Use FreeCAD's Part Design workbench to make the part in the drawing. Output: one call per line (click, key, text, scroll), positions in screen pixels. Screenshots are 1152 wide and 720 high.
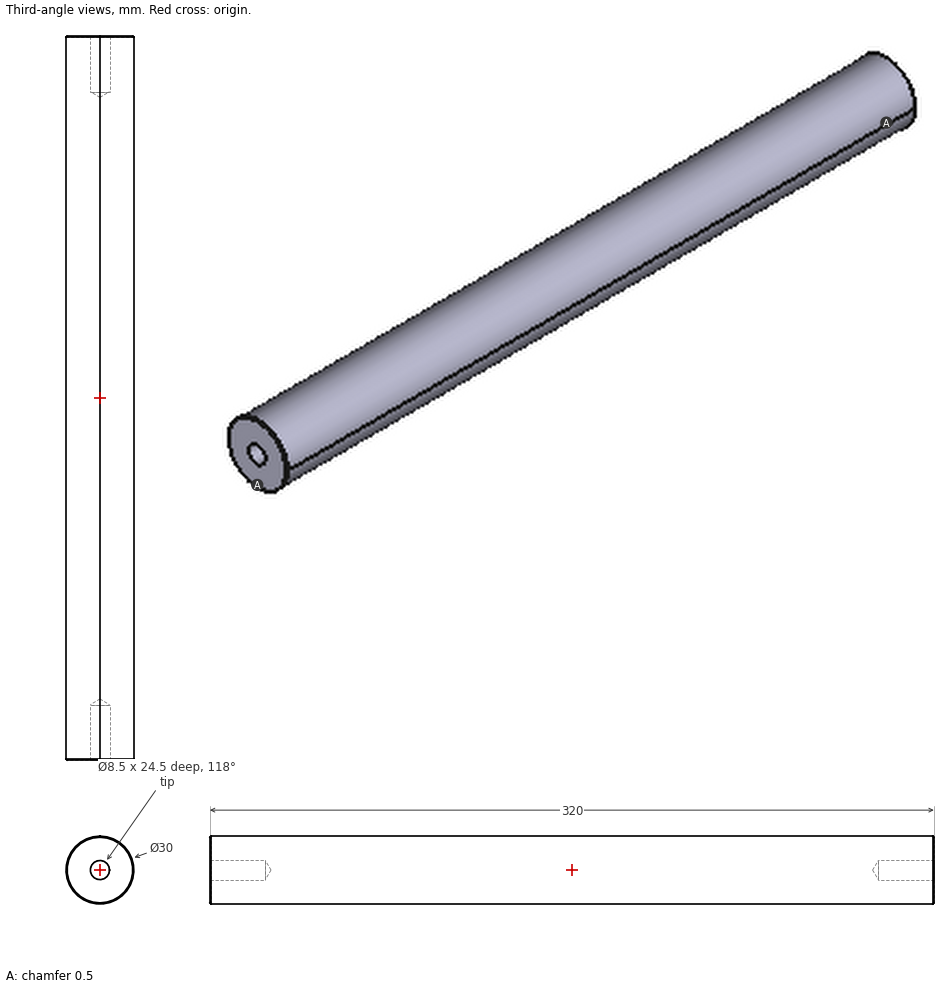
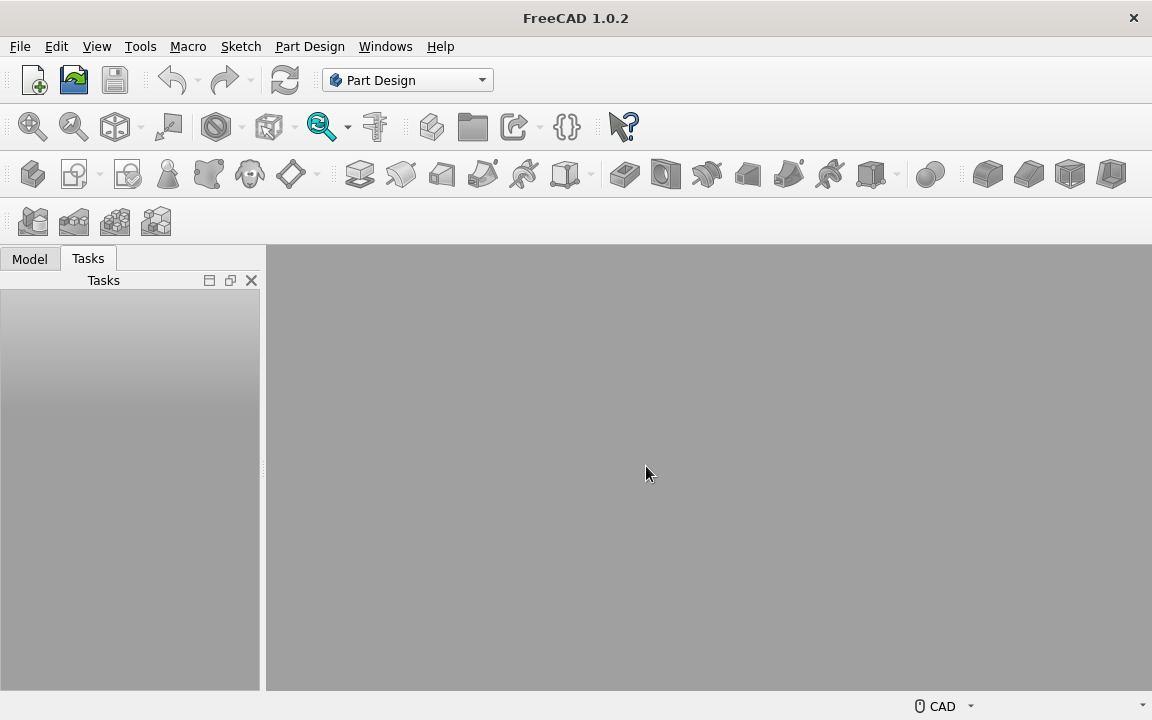
key(ctrl+n)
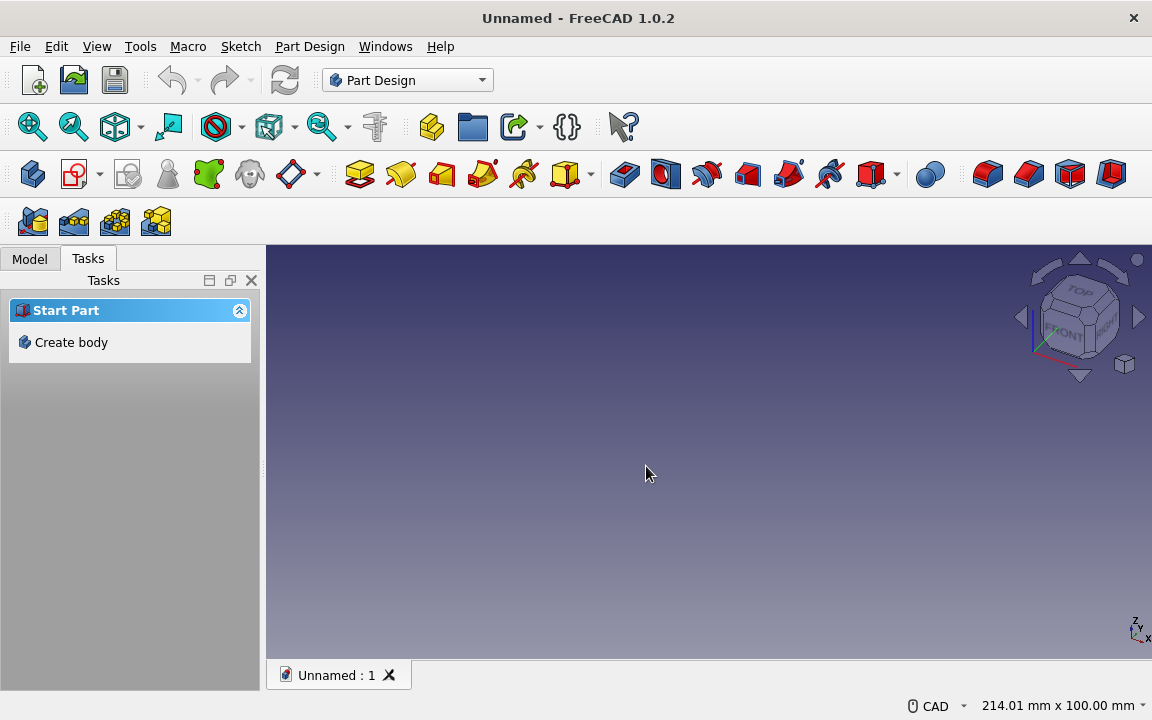
click(74, 174)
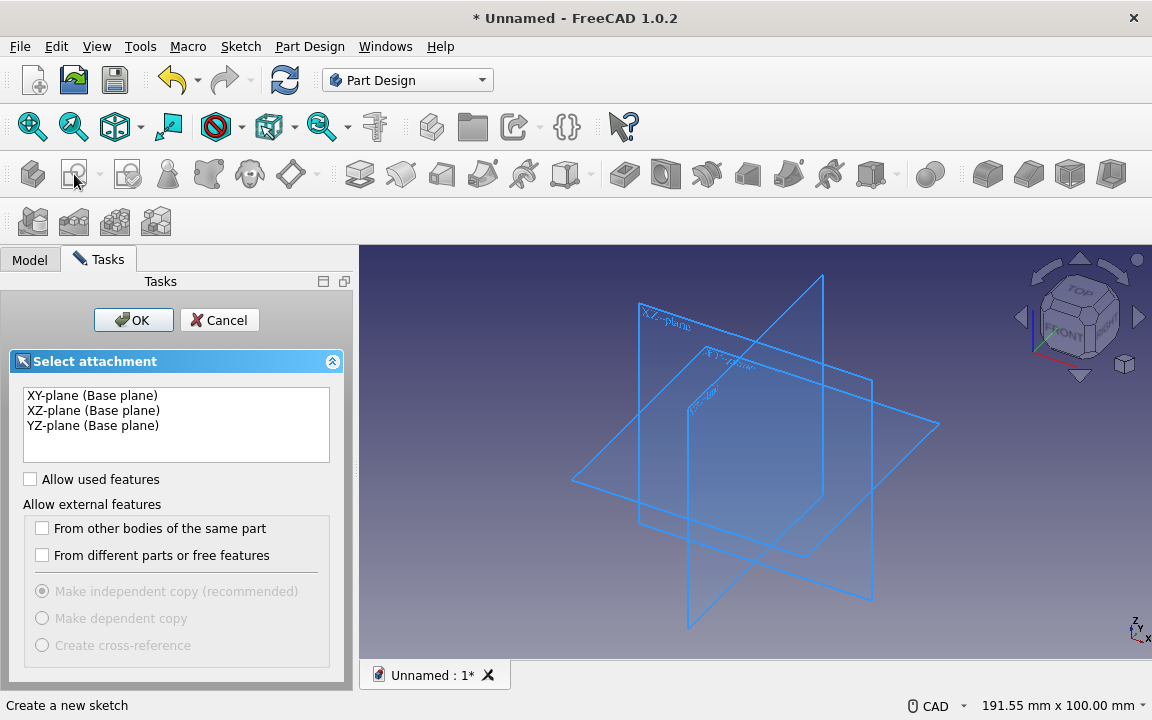
click(84, 410)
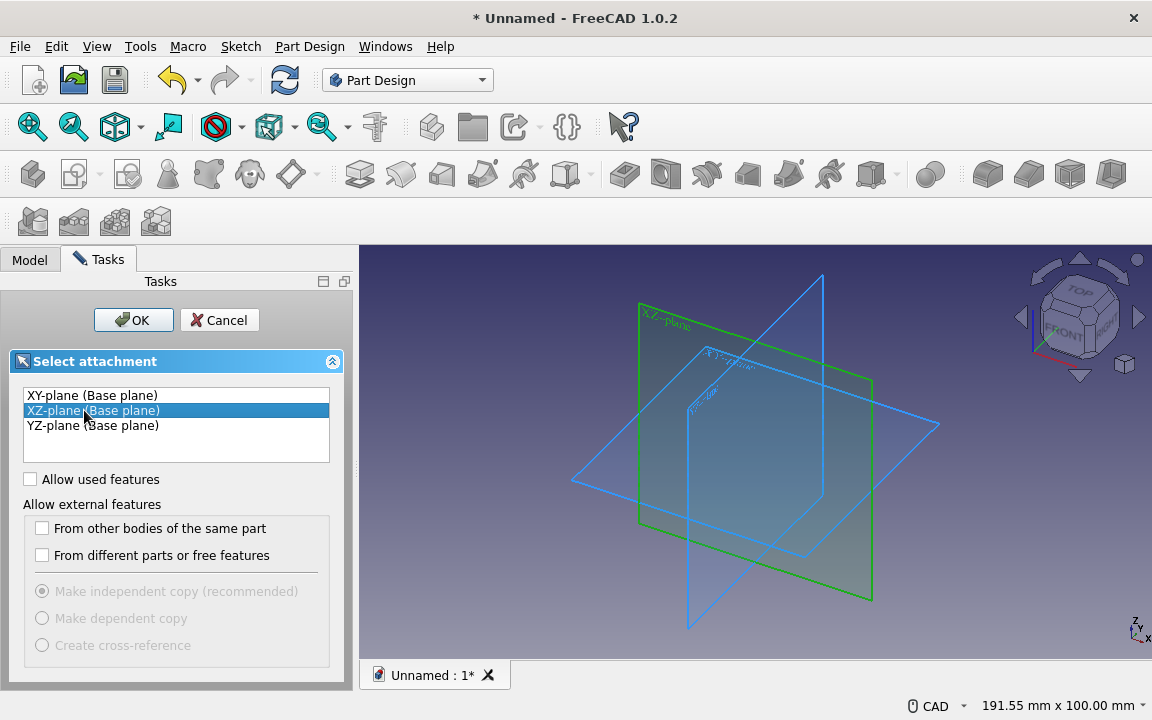
click(134, 320)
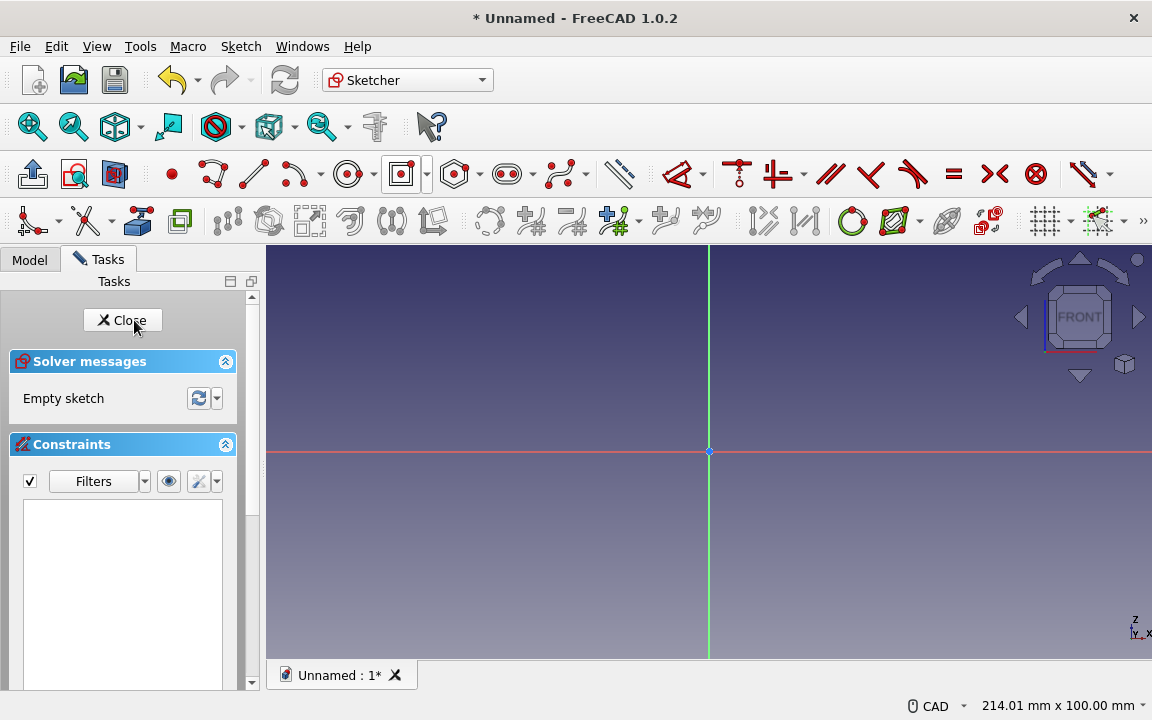
scroll(765, 452, up, 4)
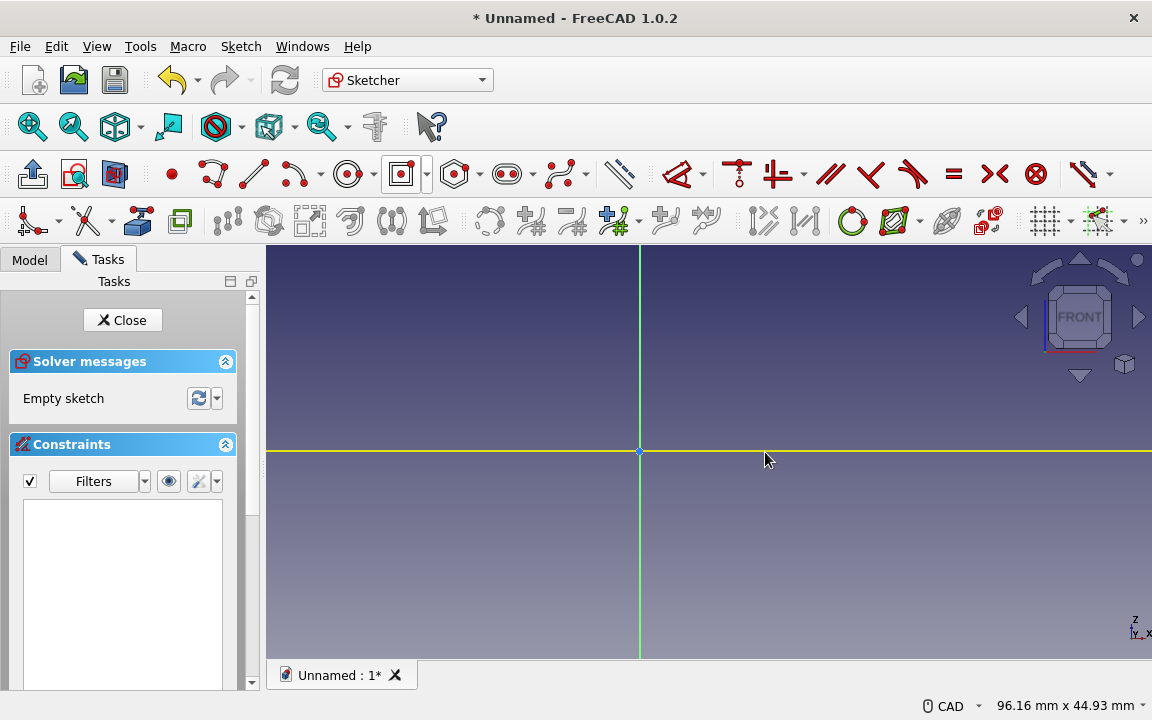
key(g)
key(c)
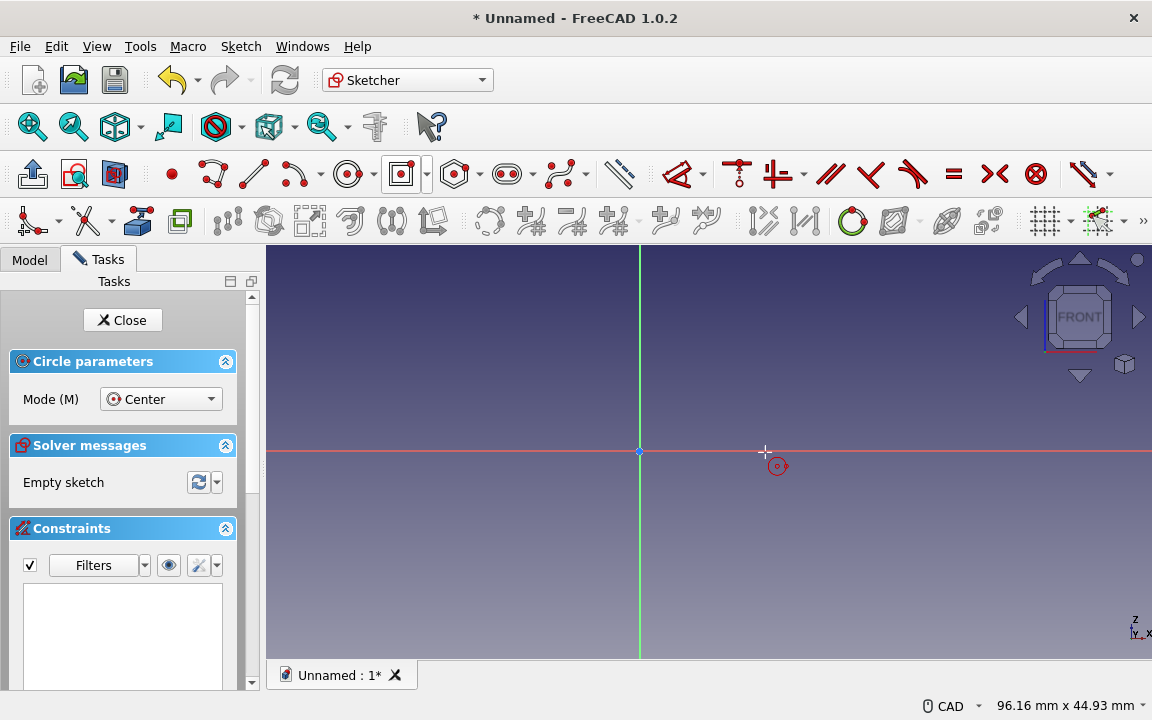
click(640, 451)
click(737, 354)
key(Escape)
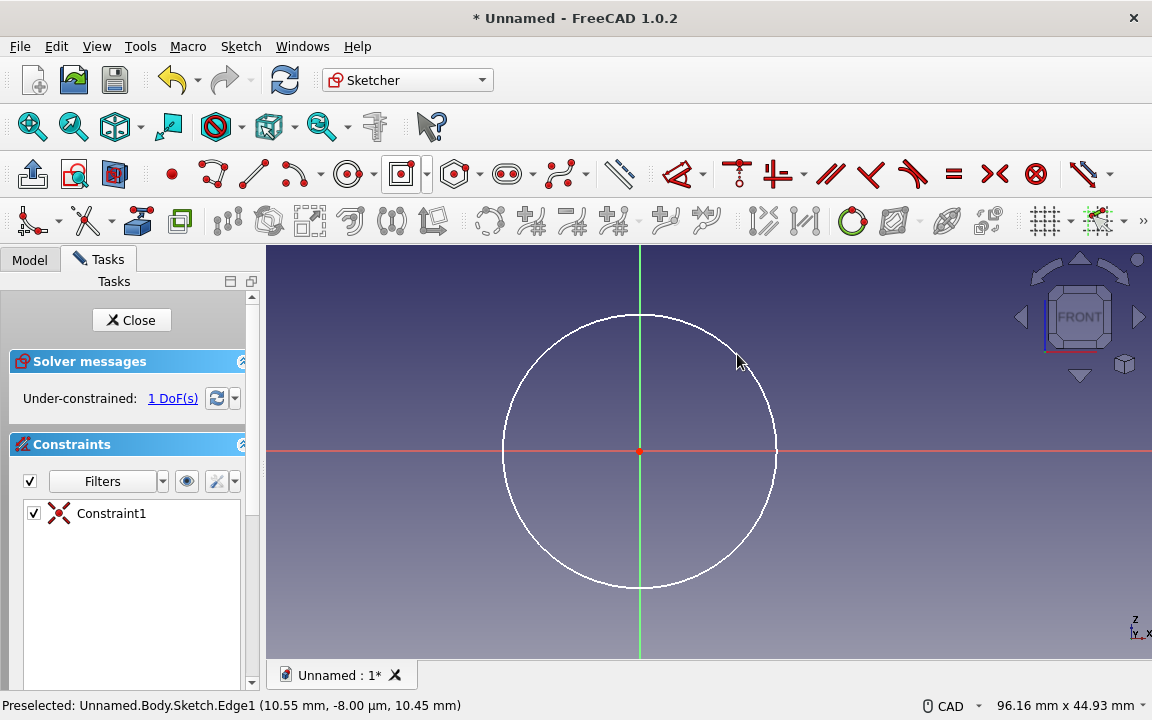
click(736, 354)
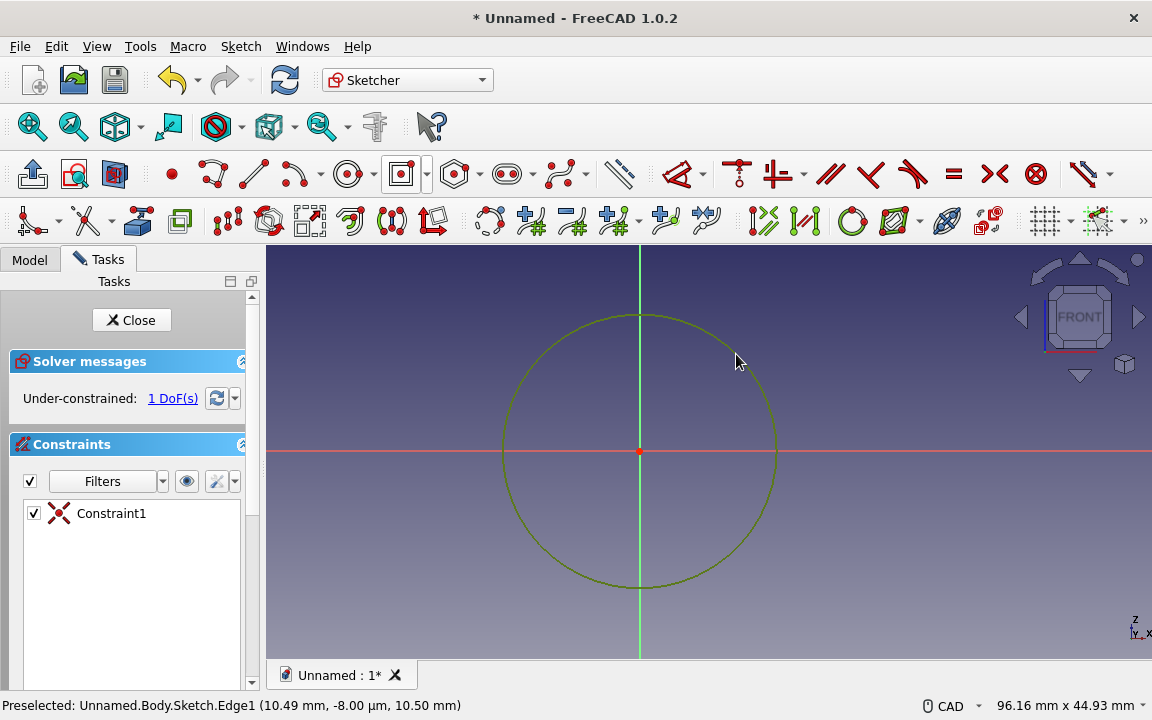
key(k)
key(o)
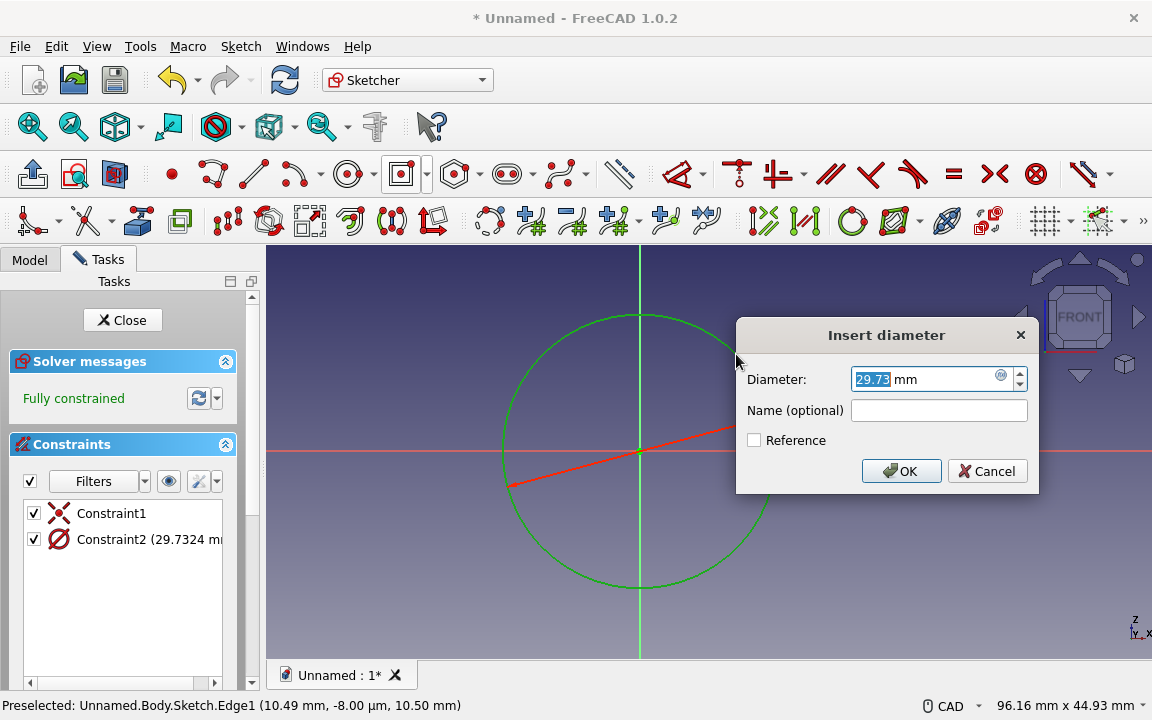
text(30)
key(Return)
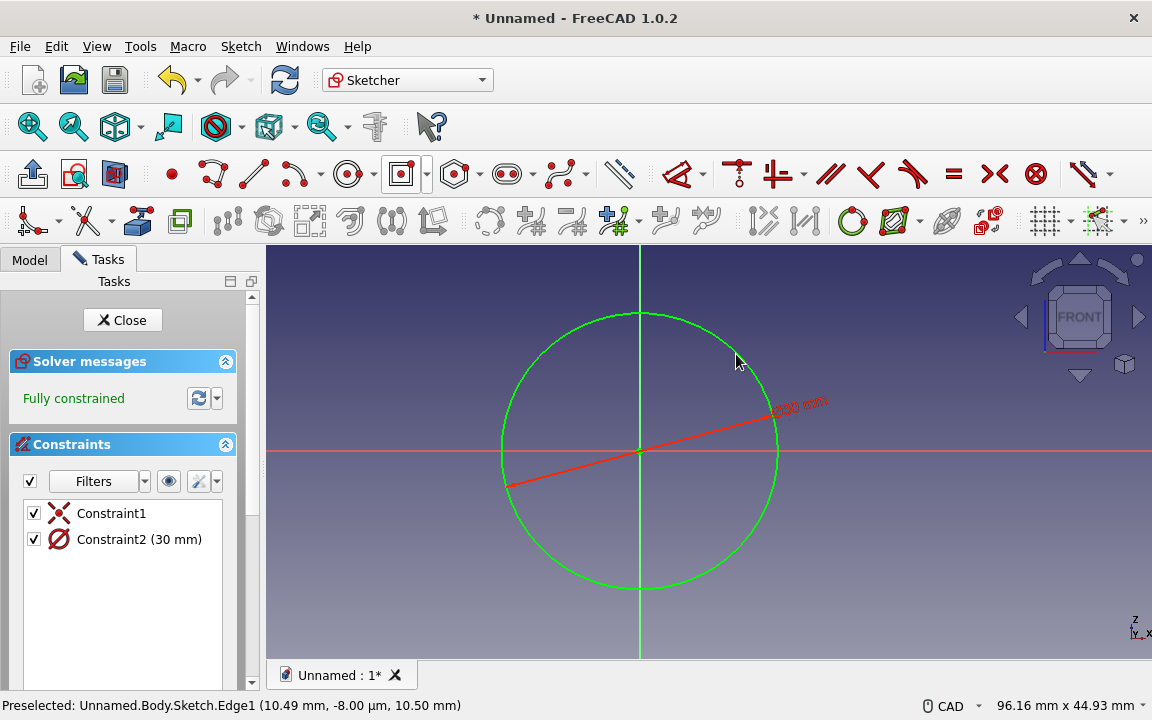
click(123, 320)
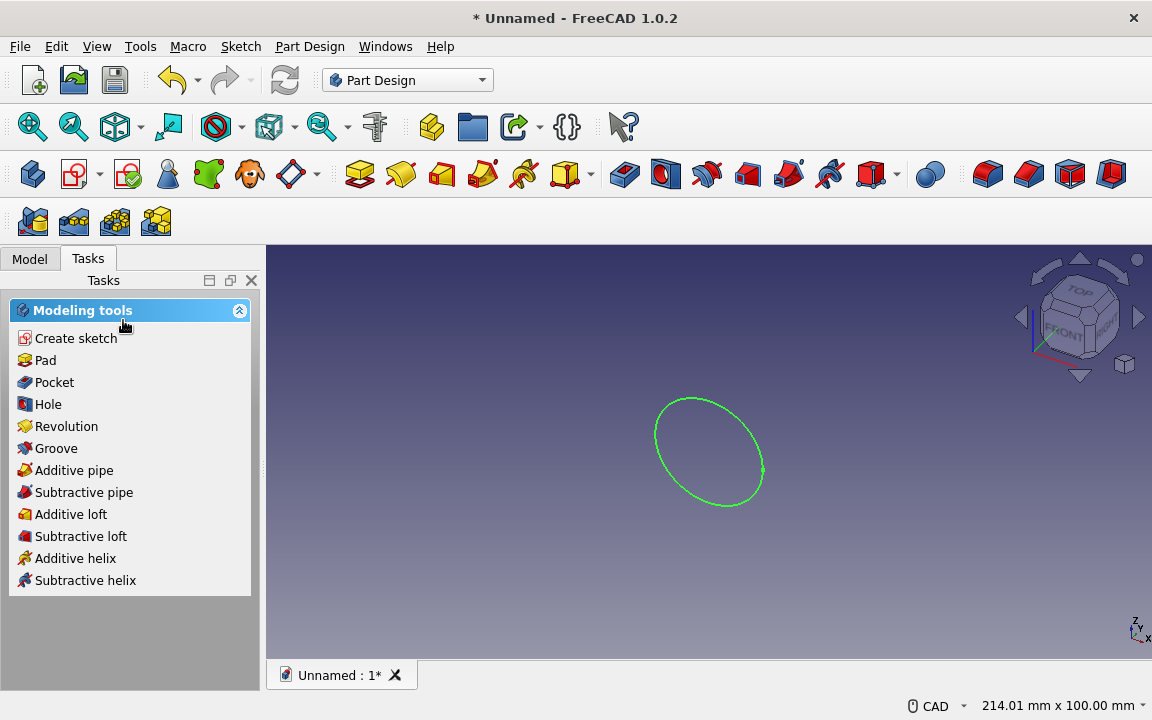
click(360, 174)